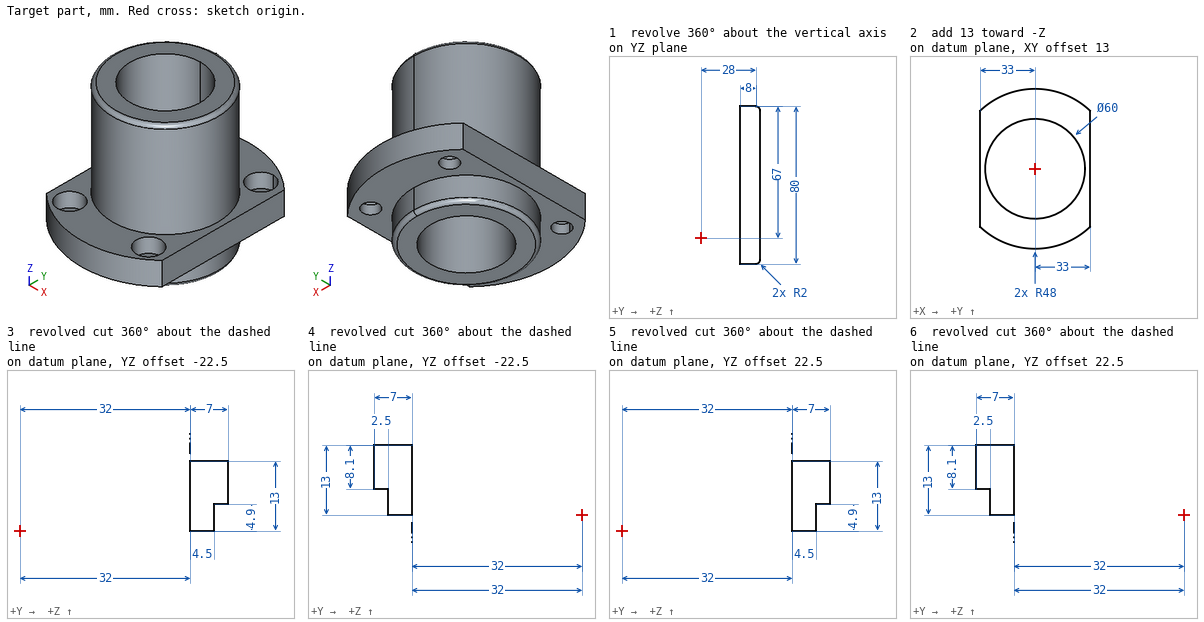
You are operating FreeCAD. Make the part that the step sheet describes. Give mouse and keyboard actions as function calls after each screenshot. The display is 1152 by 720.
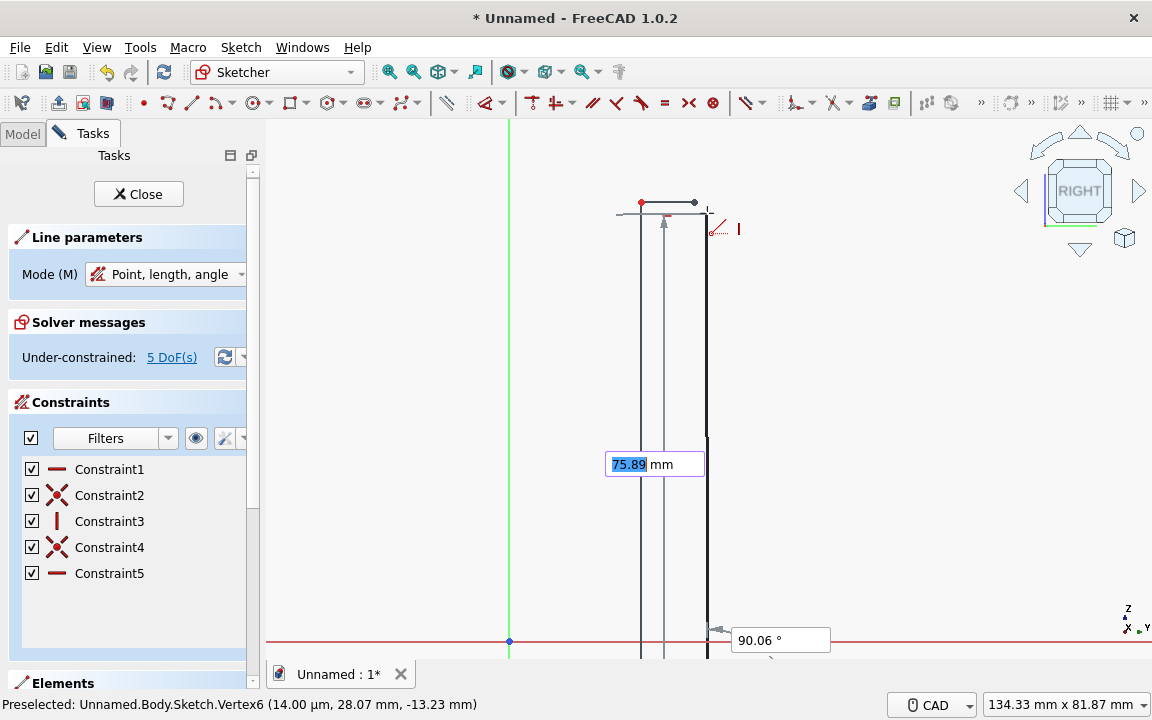
click(707, 213)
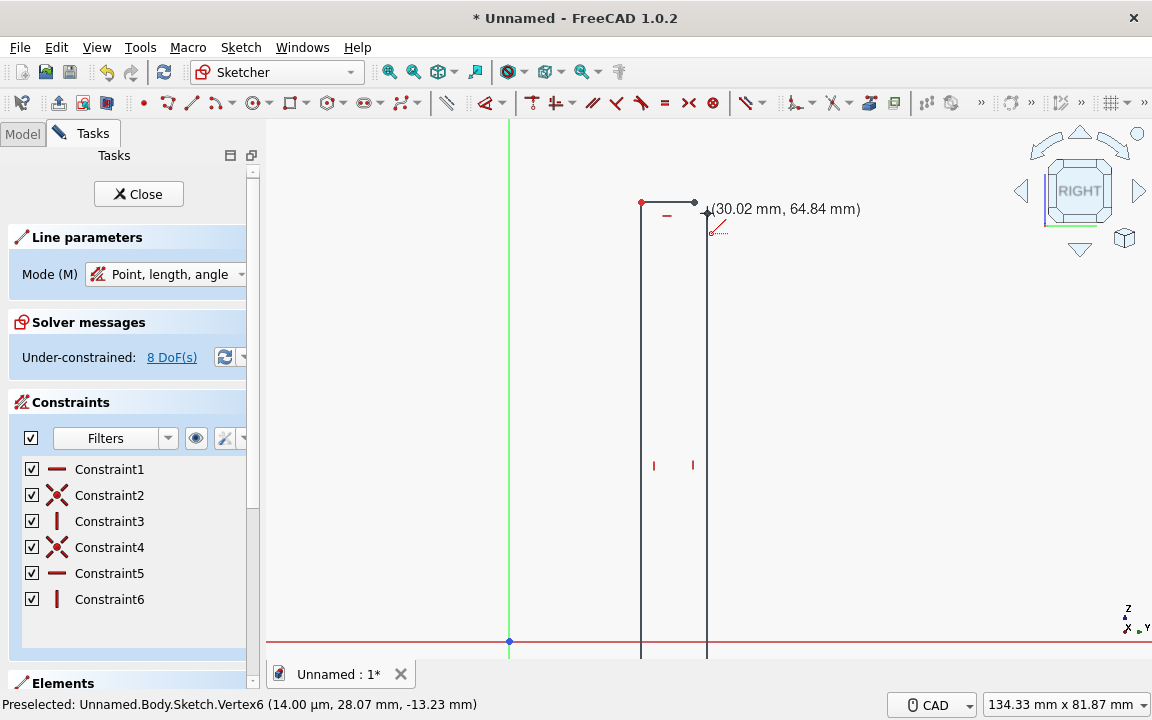
click(234, 104)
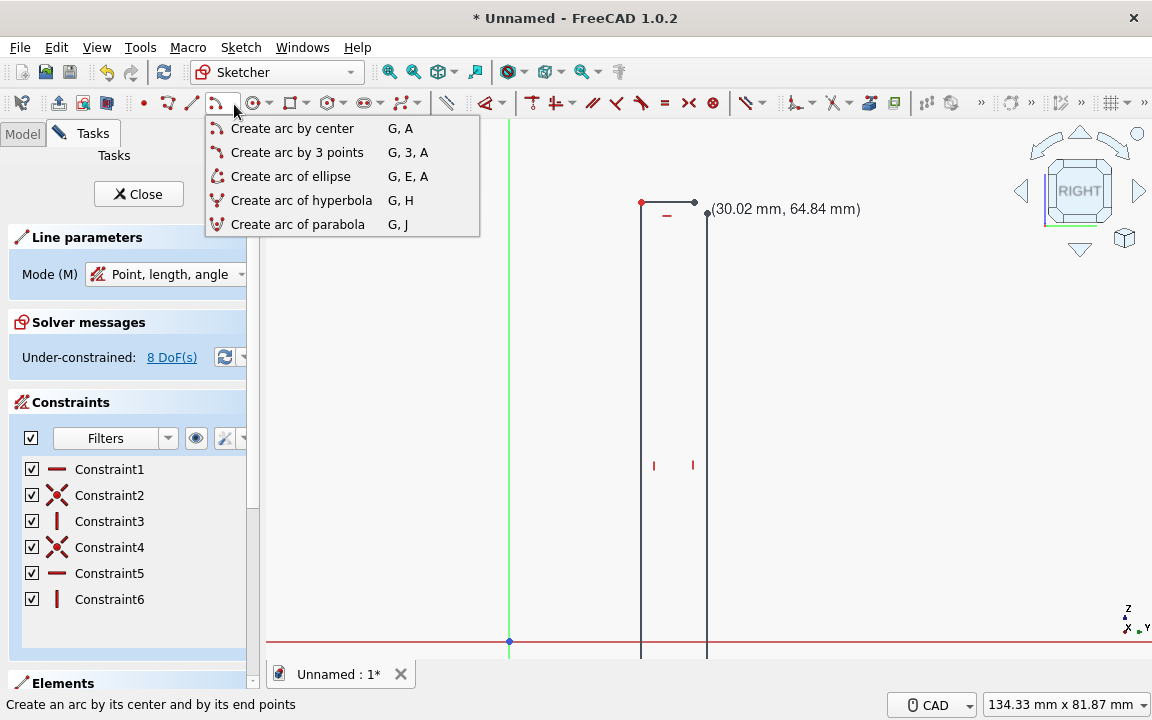
click(342, 152)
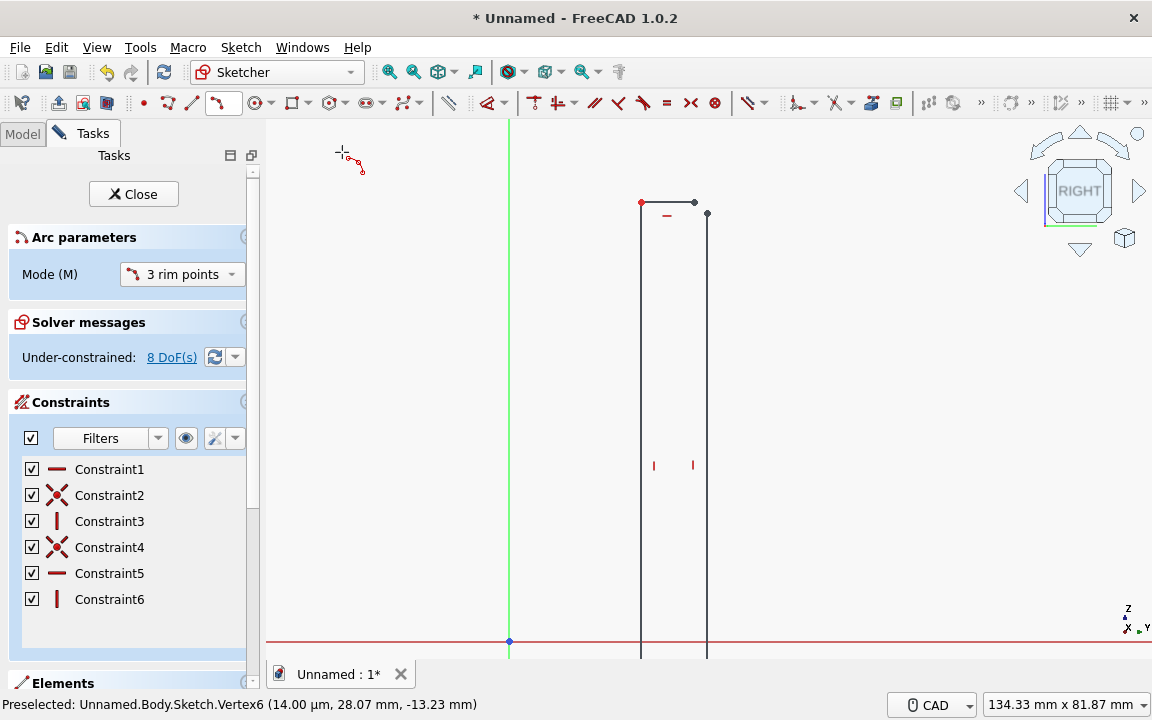
scroll(707, 237, down, 2)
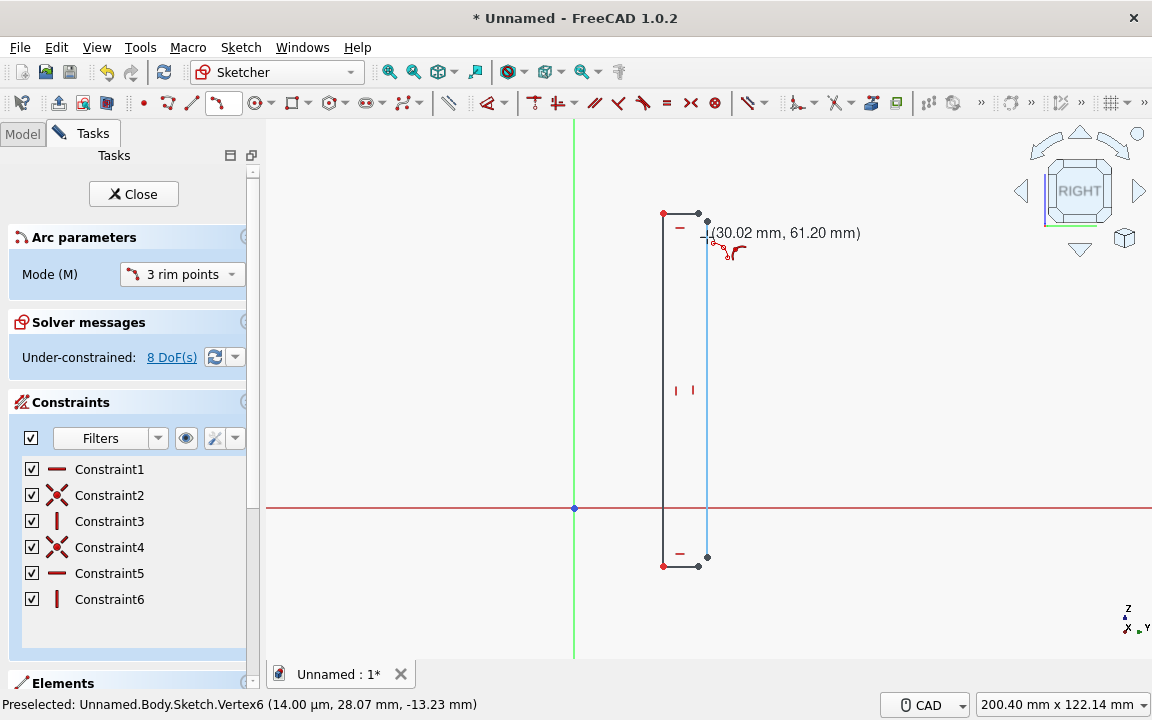
scroll(698, 566, up, 2)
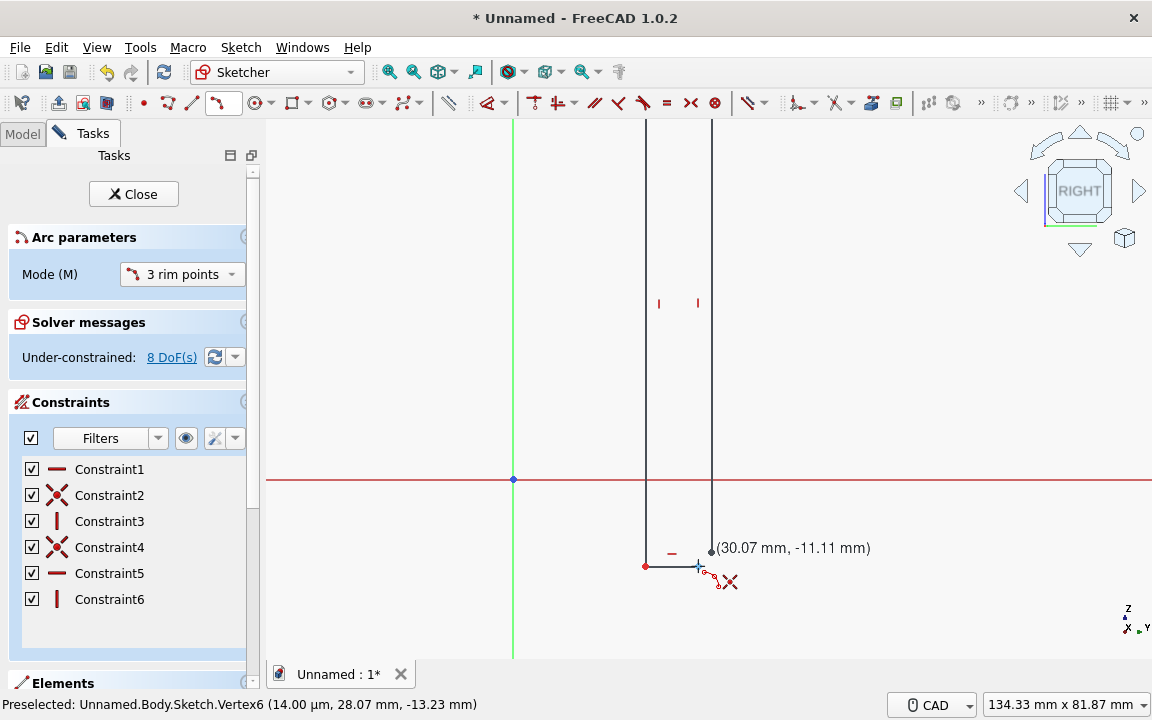
click(699, 567)
click(712, 553)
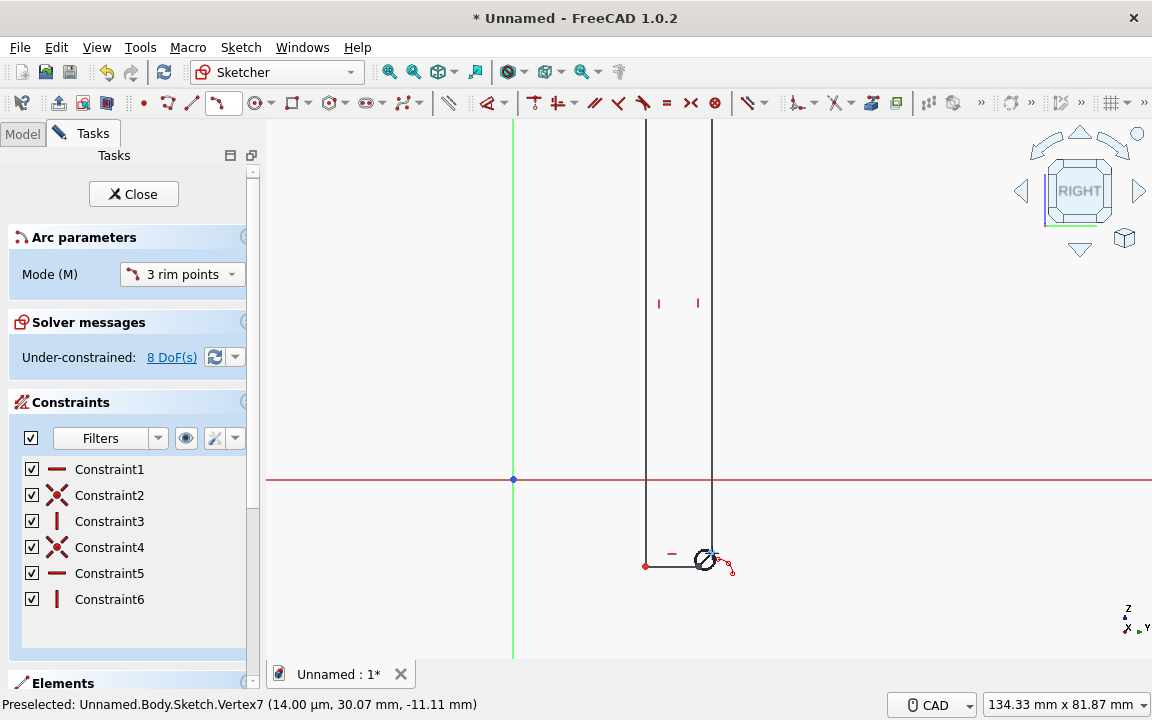
scroll(707, 561, up, 8)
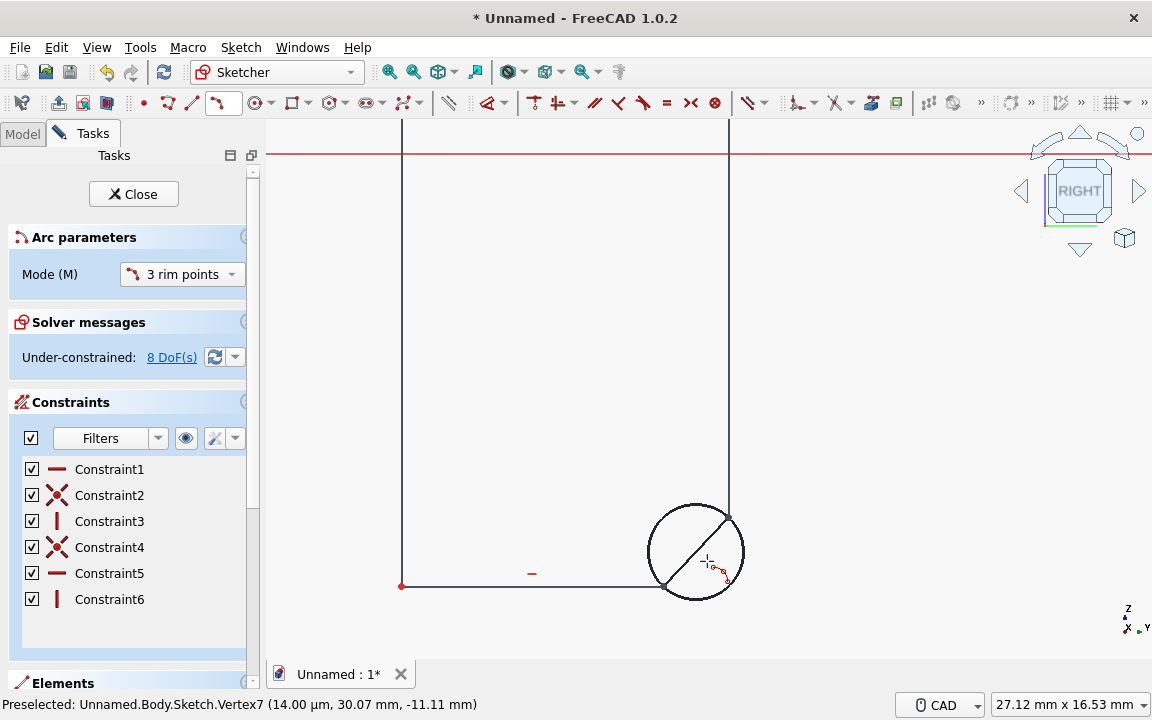
click(707, 560)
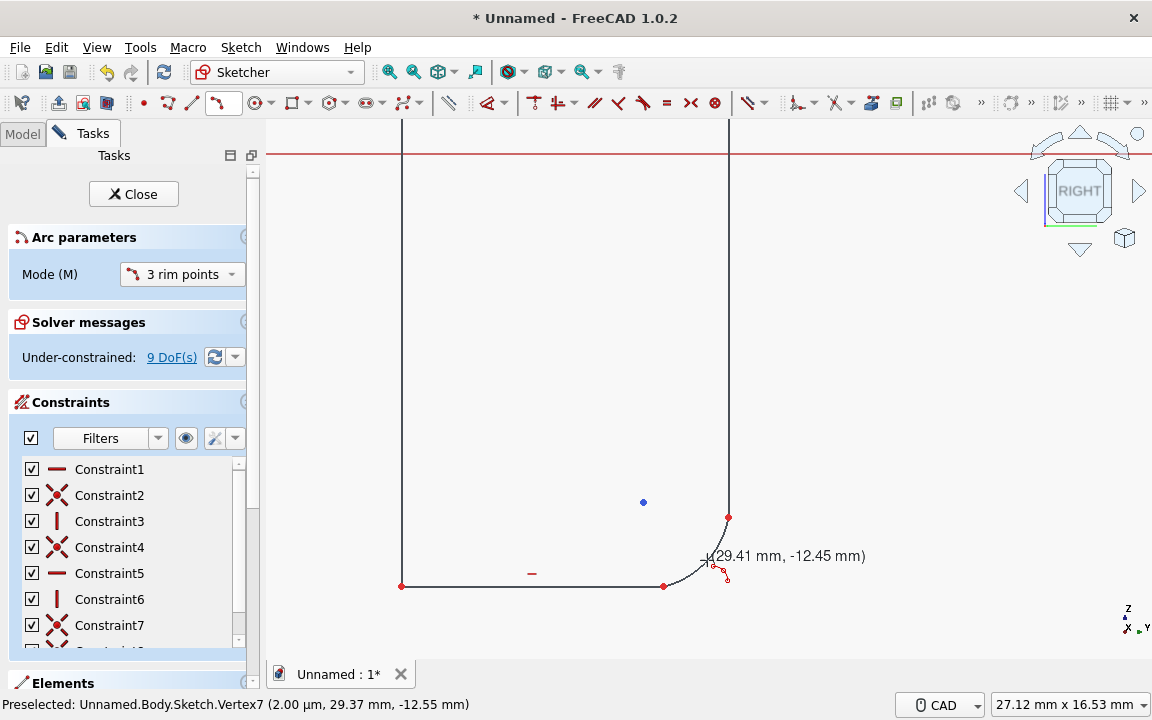
scroll(704, 564, down, 10)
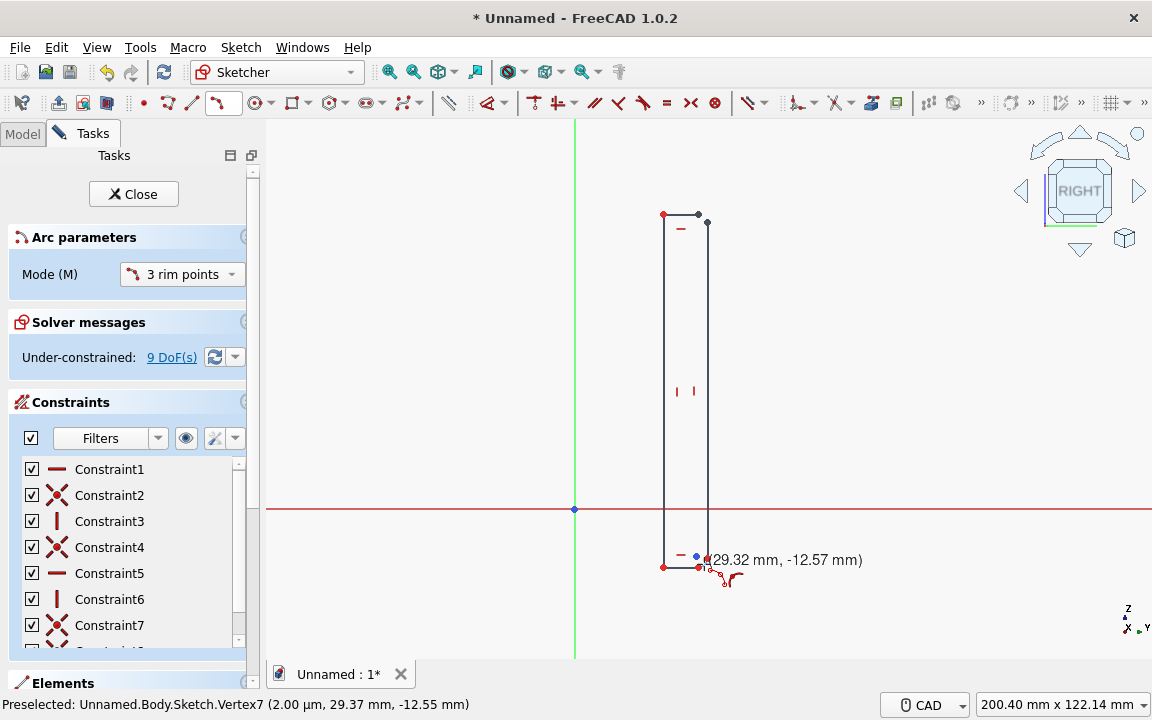
scroll(707, 222, up, 2)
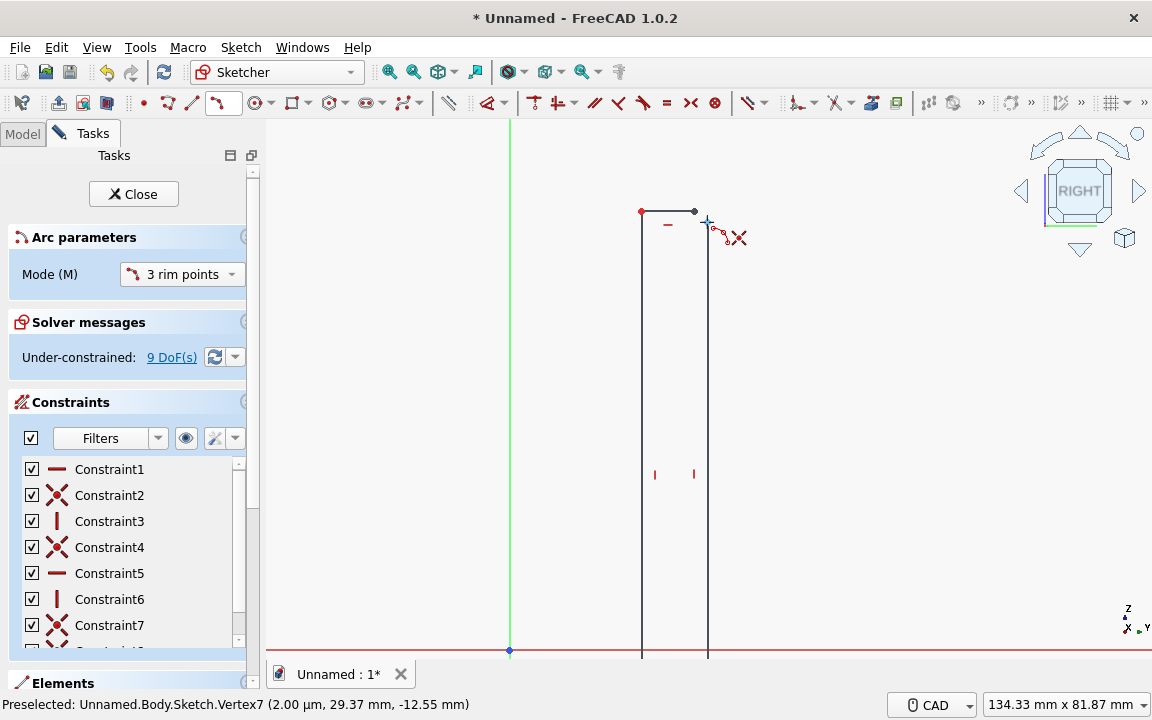
click(708, 223)
click(695, 211)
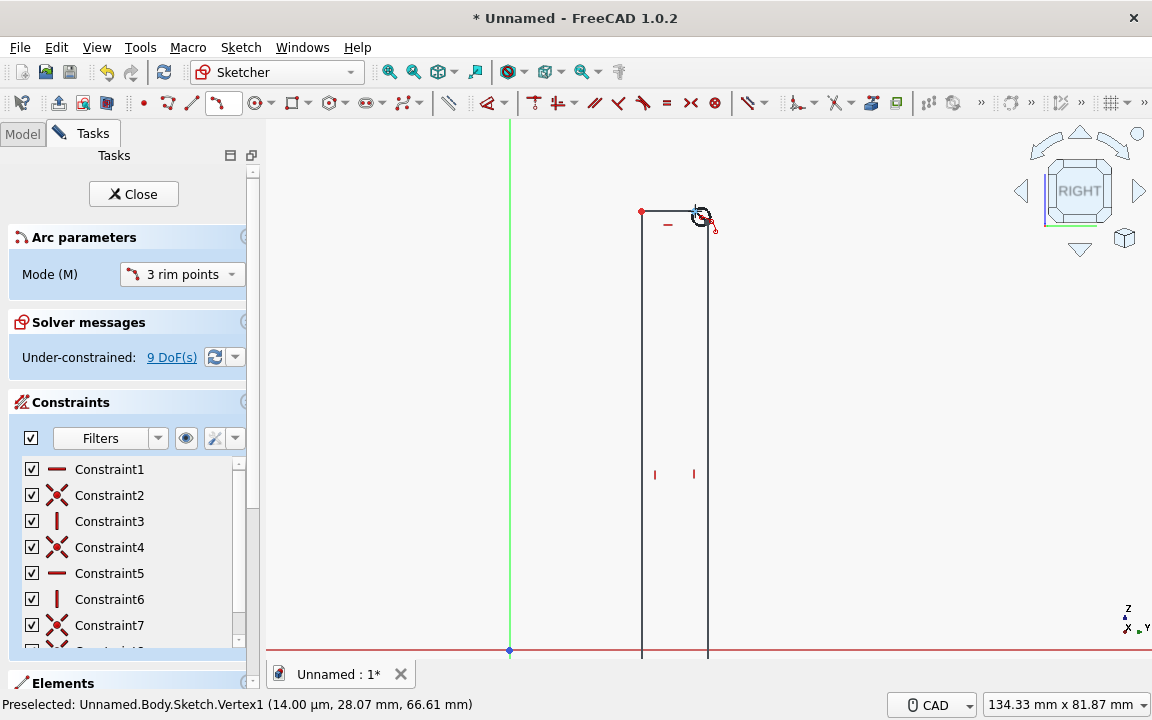
scroll(704, 212, up, 8)